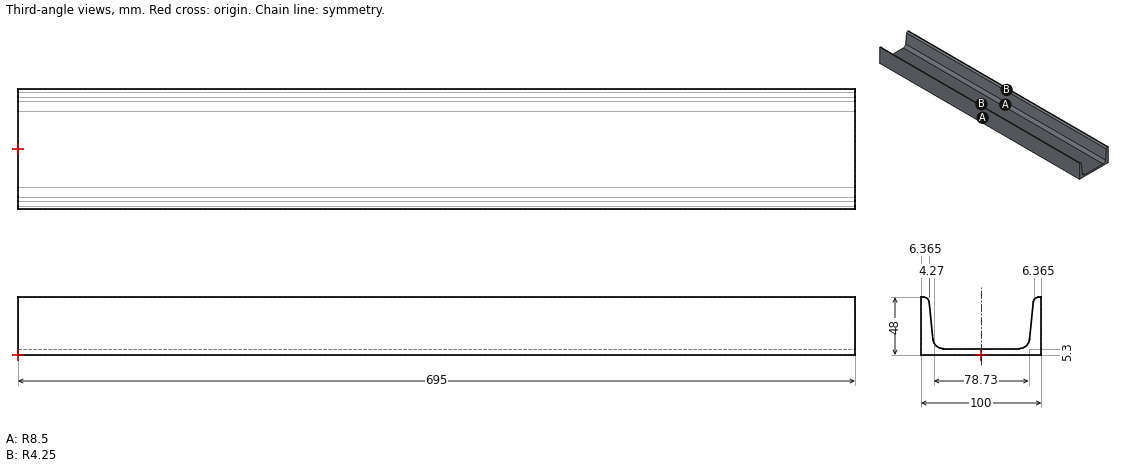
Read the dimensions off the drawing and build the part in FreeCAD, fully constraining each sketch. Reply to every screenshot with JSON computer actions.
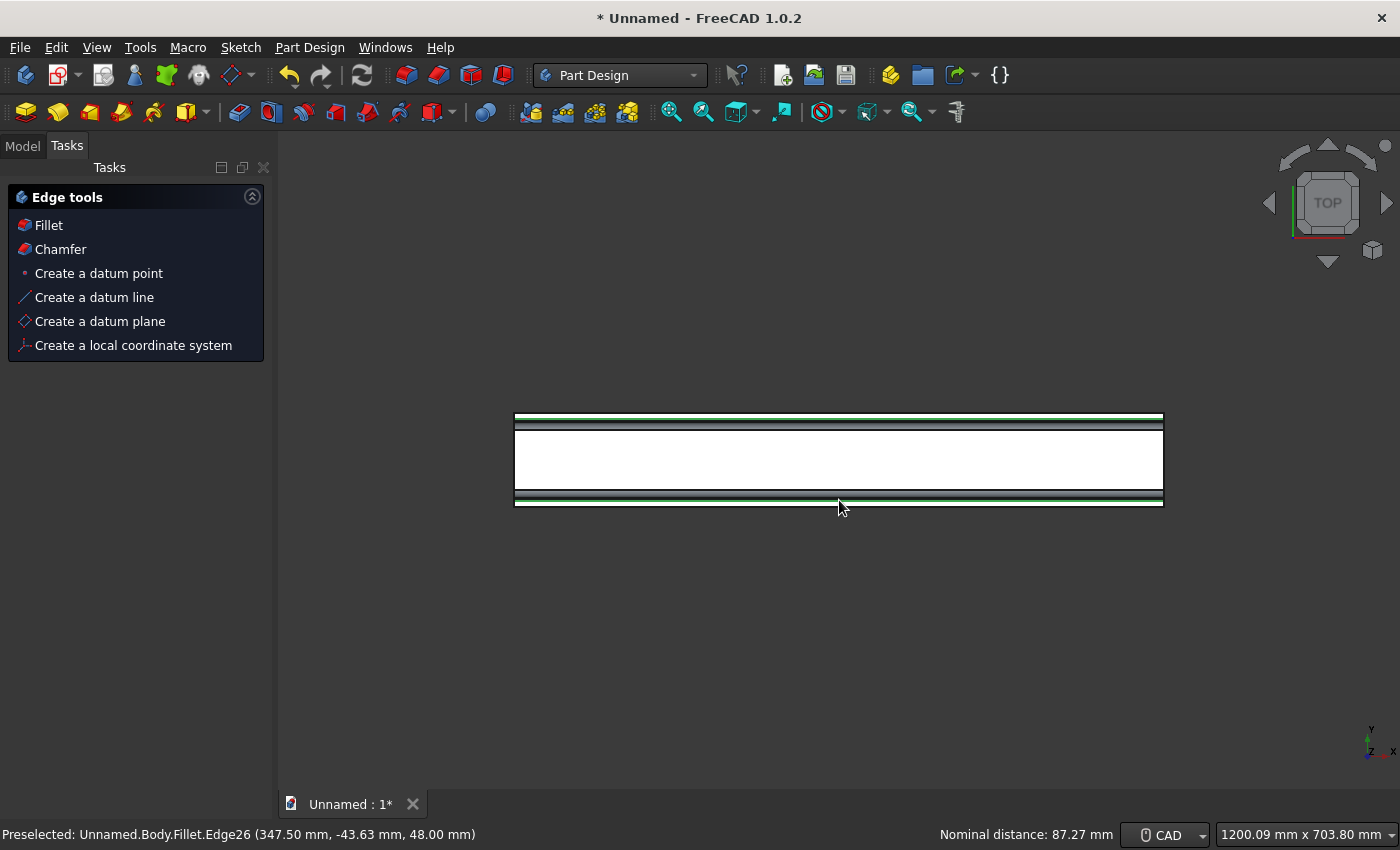
{"action": "left_click", "coordinate": [408, 76]}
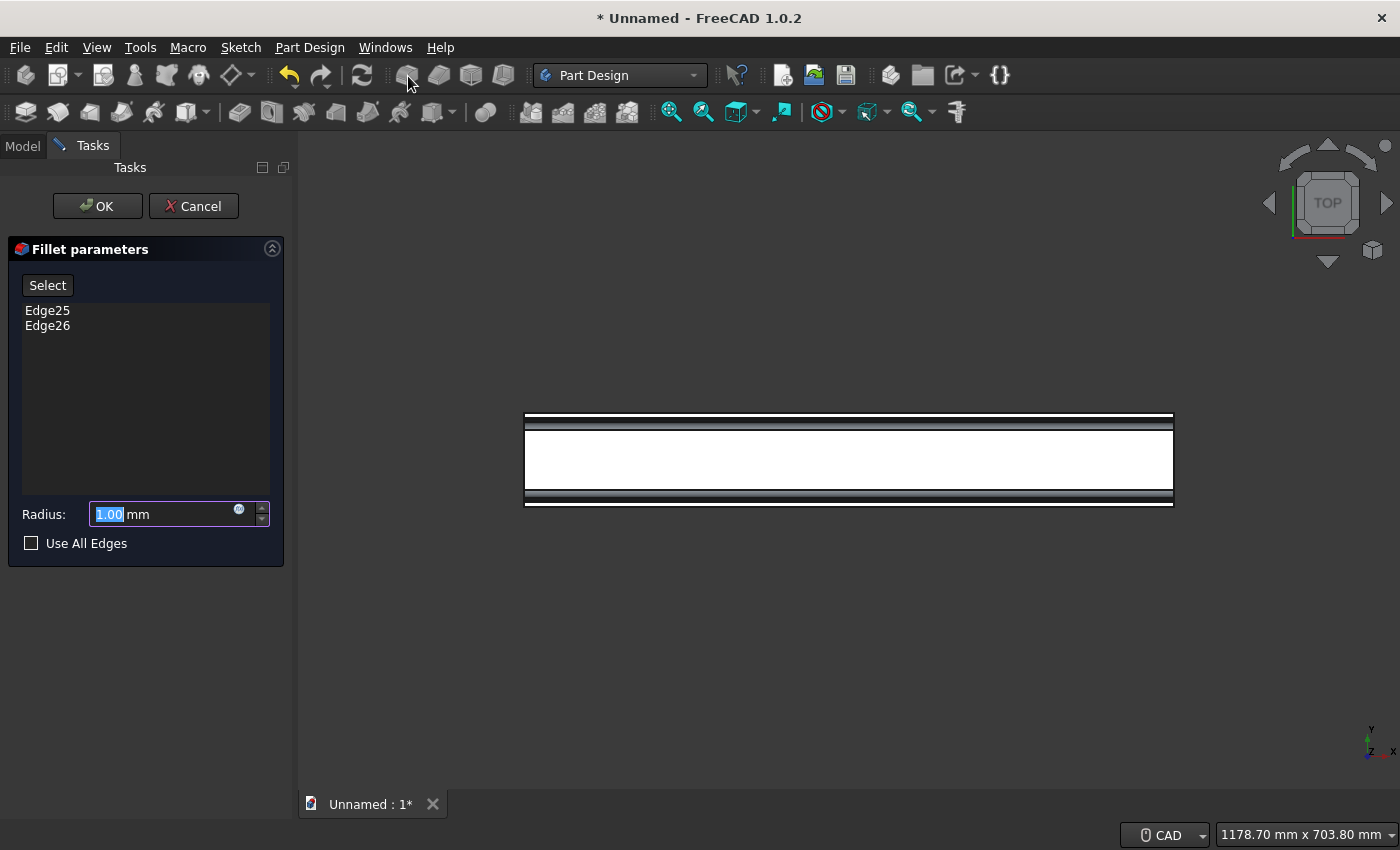
{"action": "type", "text": "4.25"}
{"action": "key", "text": "Tab"}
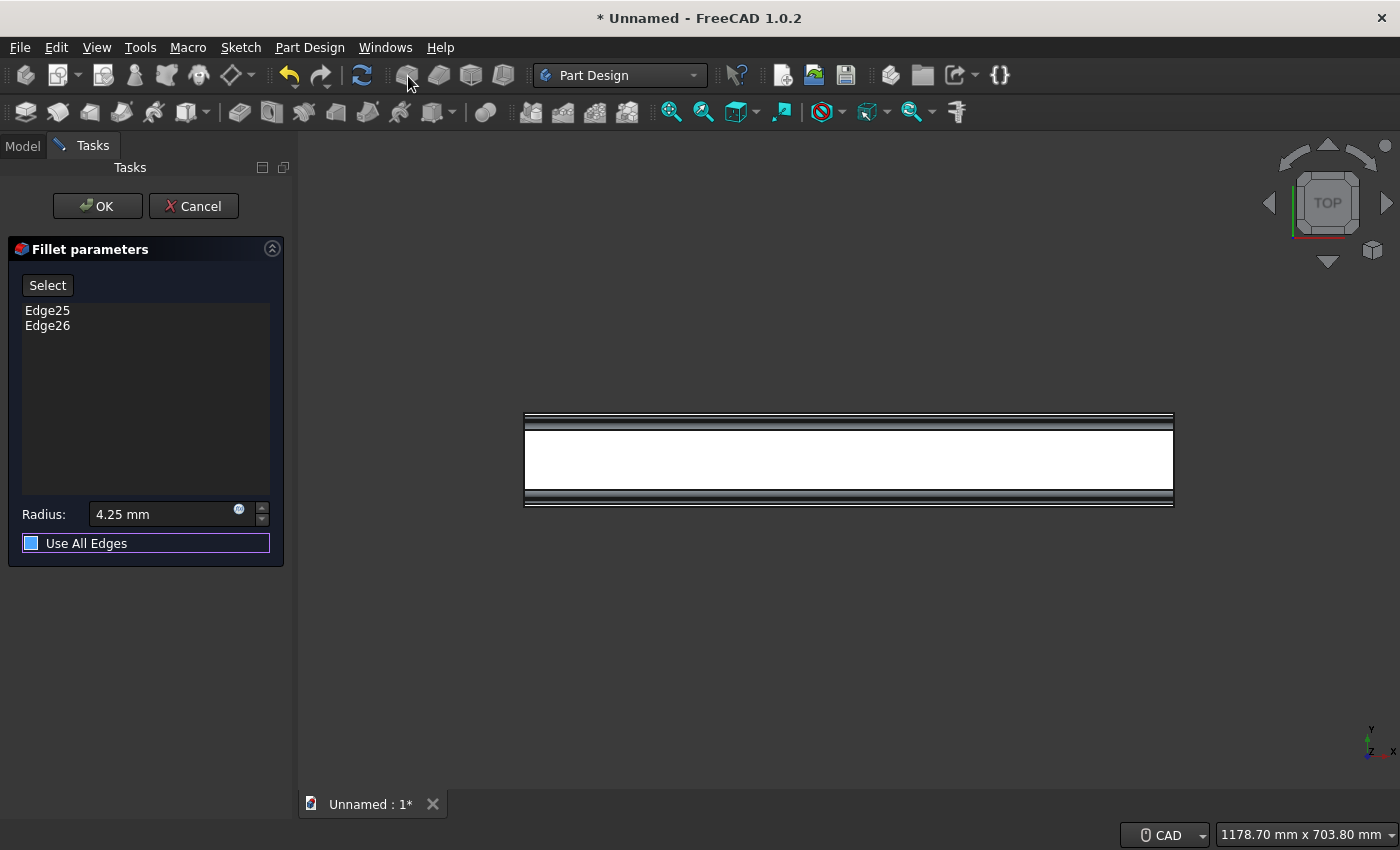
{"action": "left_click", "coordinate": [98, 206]}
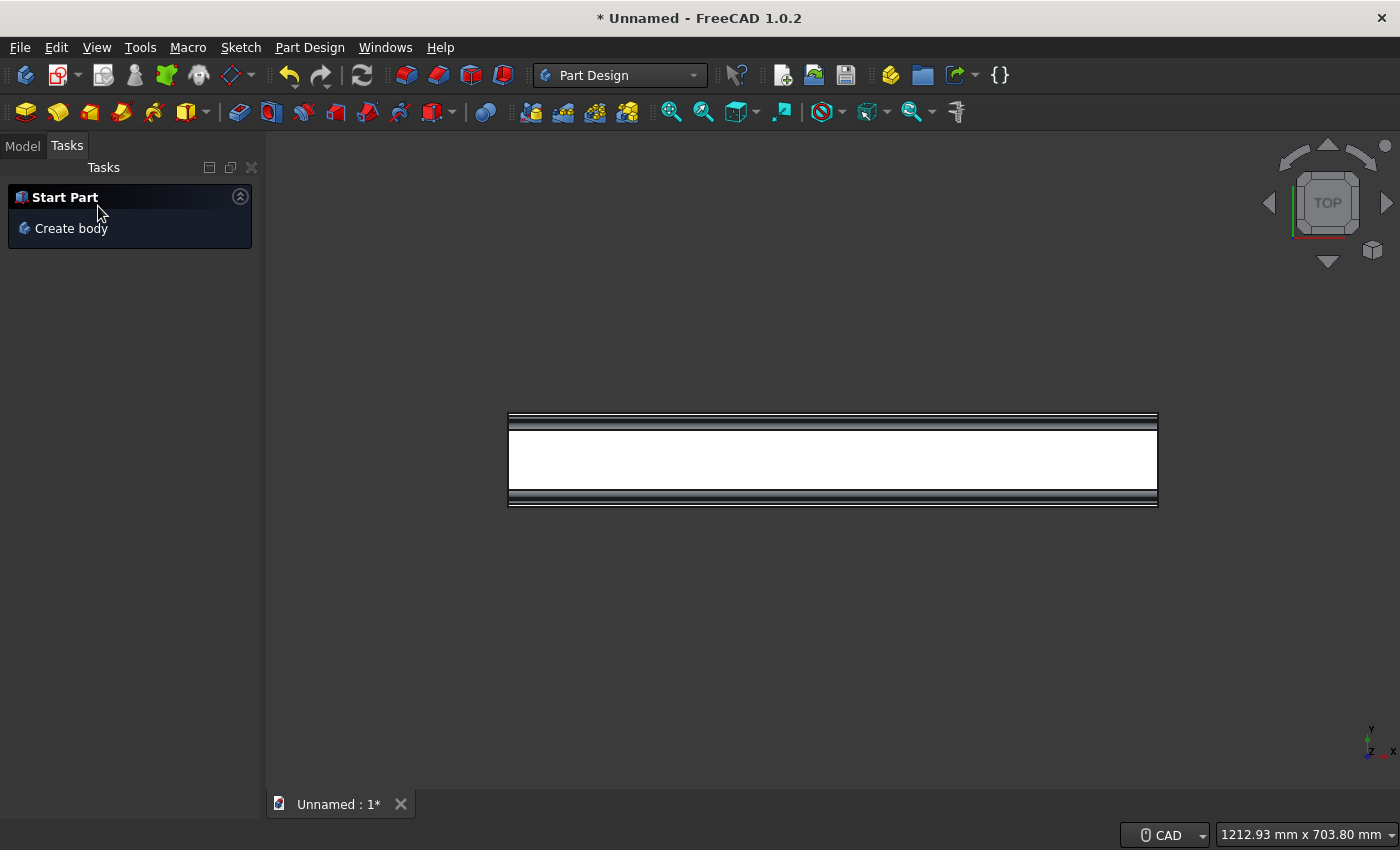
{"action": "key", "text": "0"}